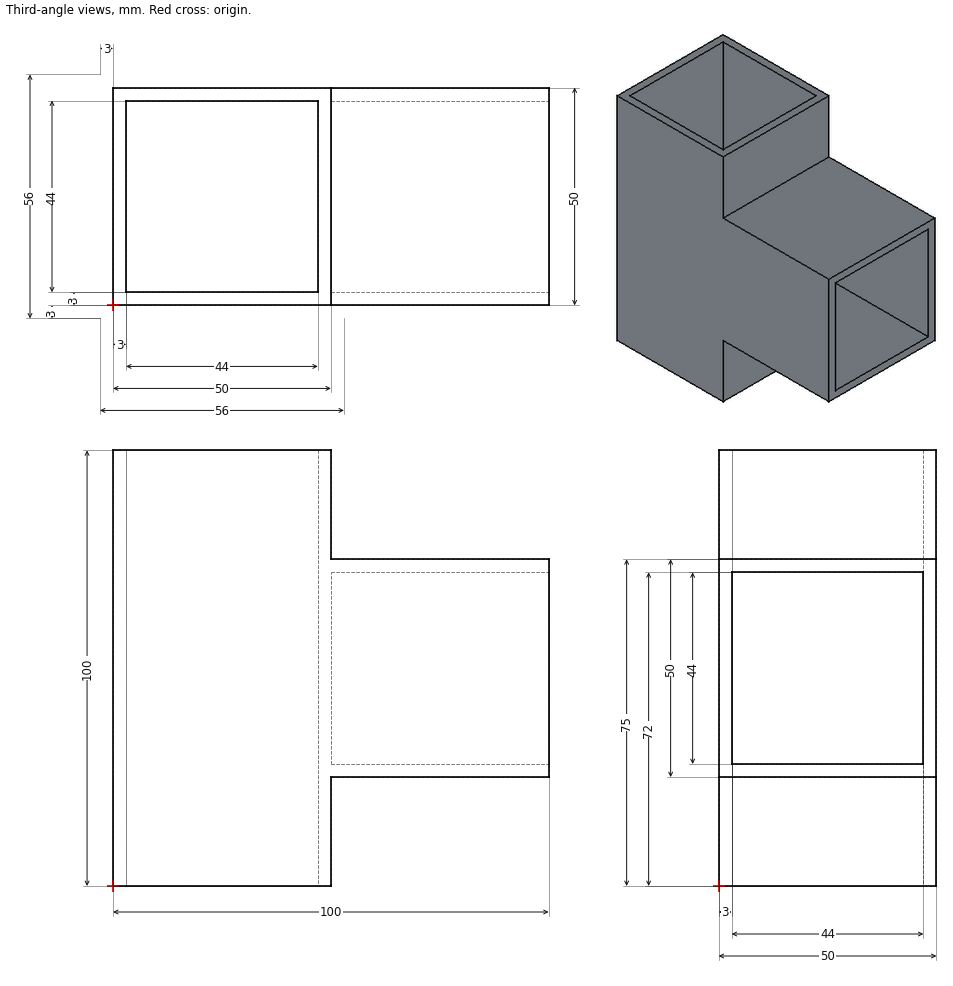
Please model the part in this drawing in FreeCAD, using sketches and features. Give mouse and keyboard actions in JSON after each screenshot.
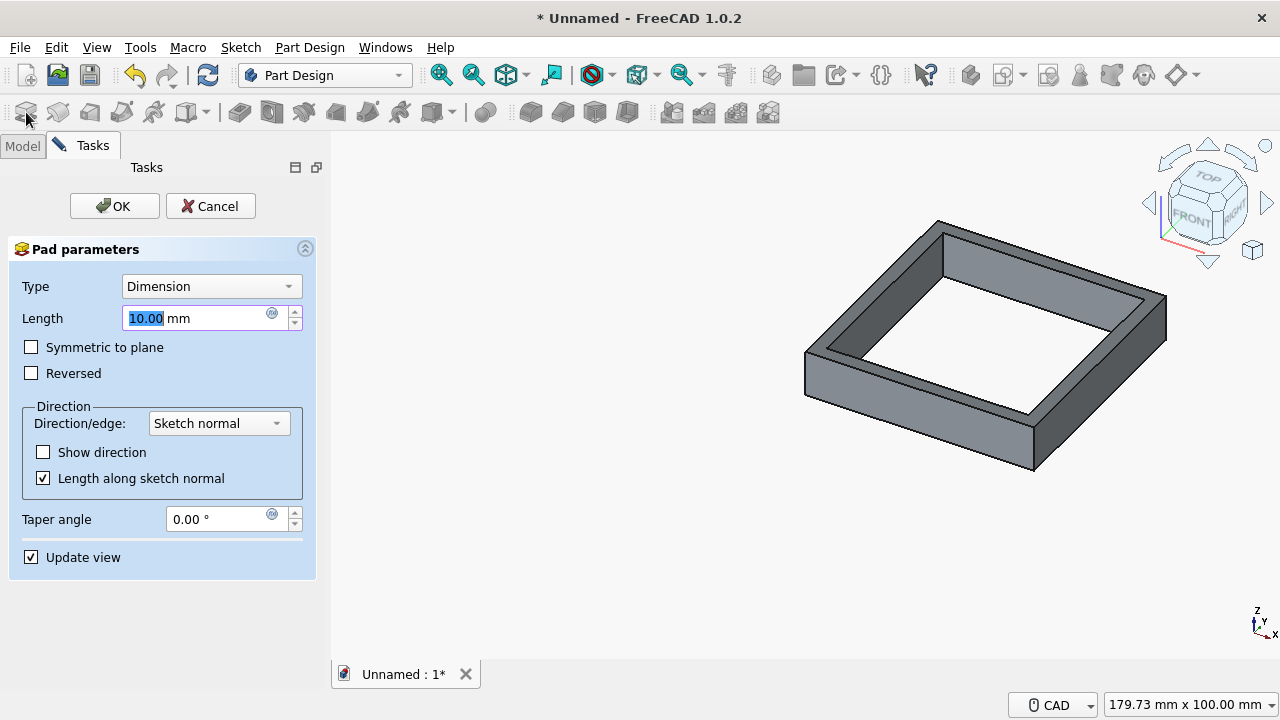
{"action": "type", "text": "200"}
{"action": "key", "text": "Tab"}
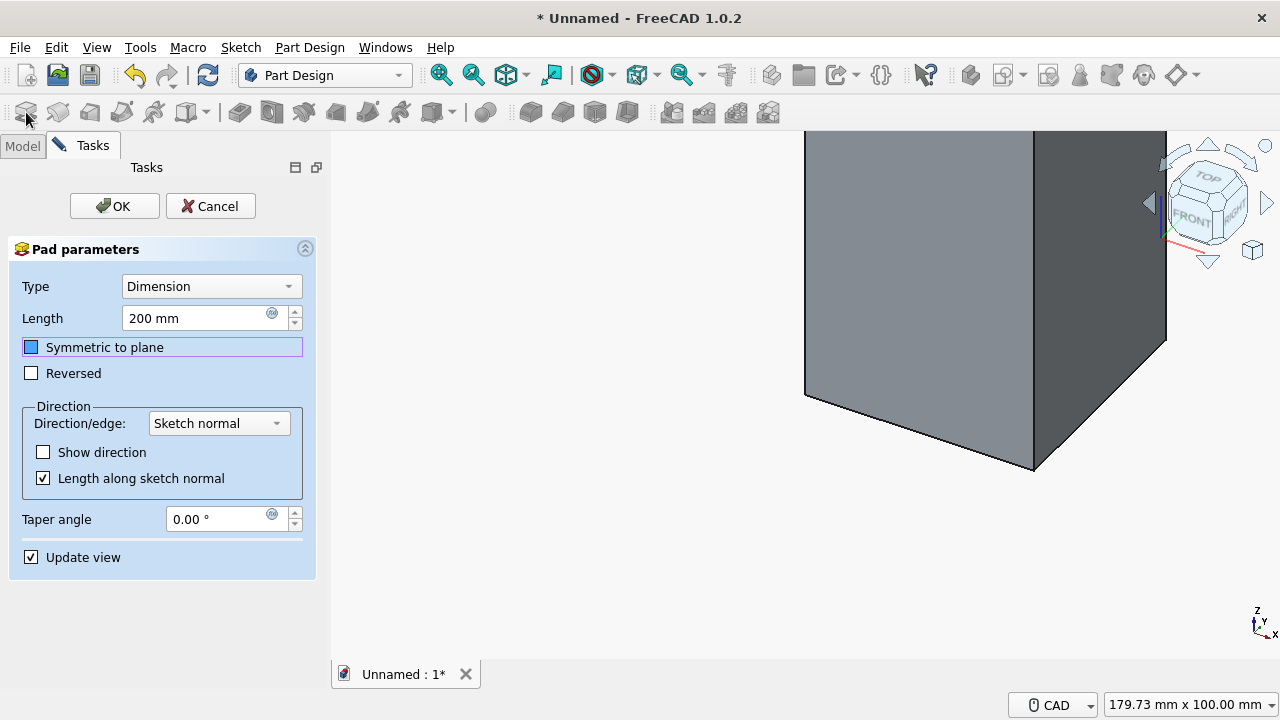
{"action": "left_click", "coordinate": [115, 206]}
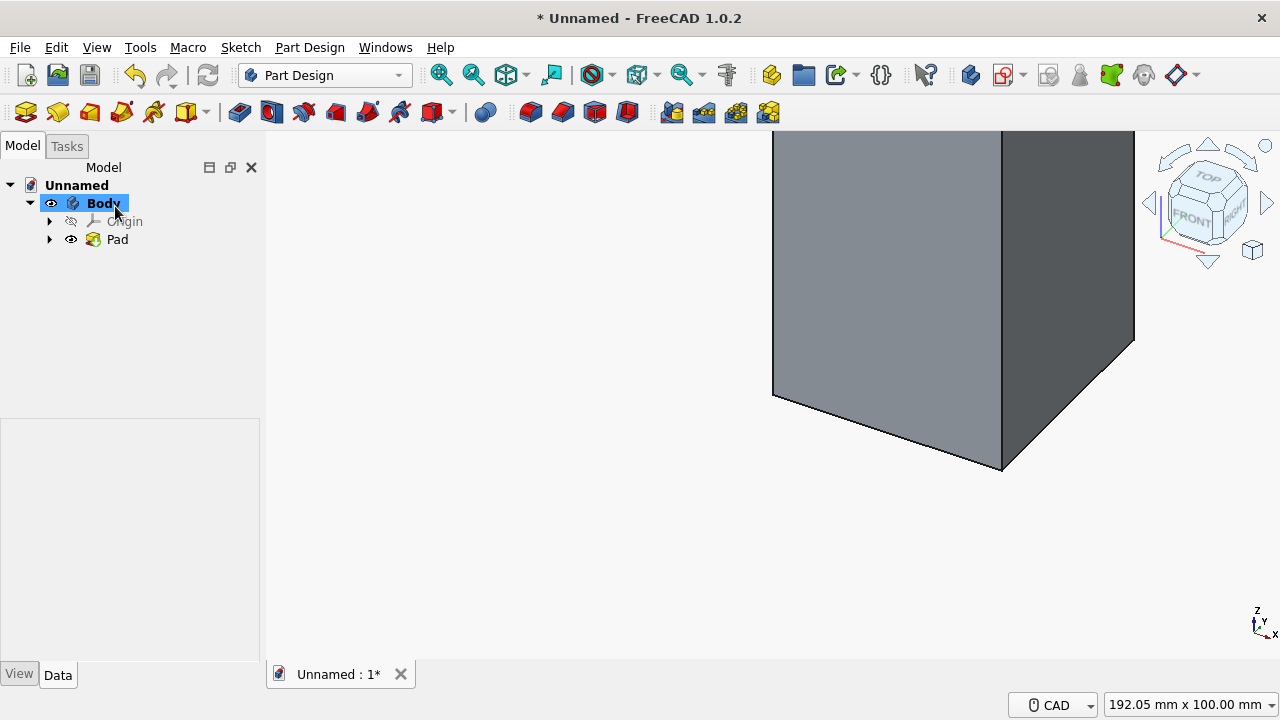
{"action": "key", "text": "v f"}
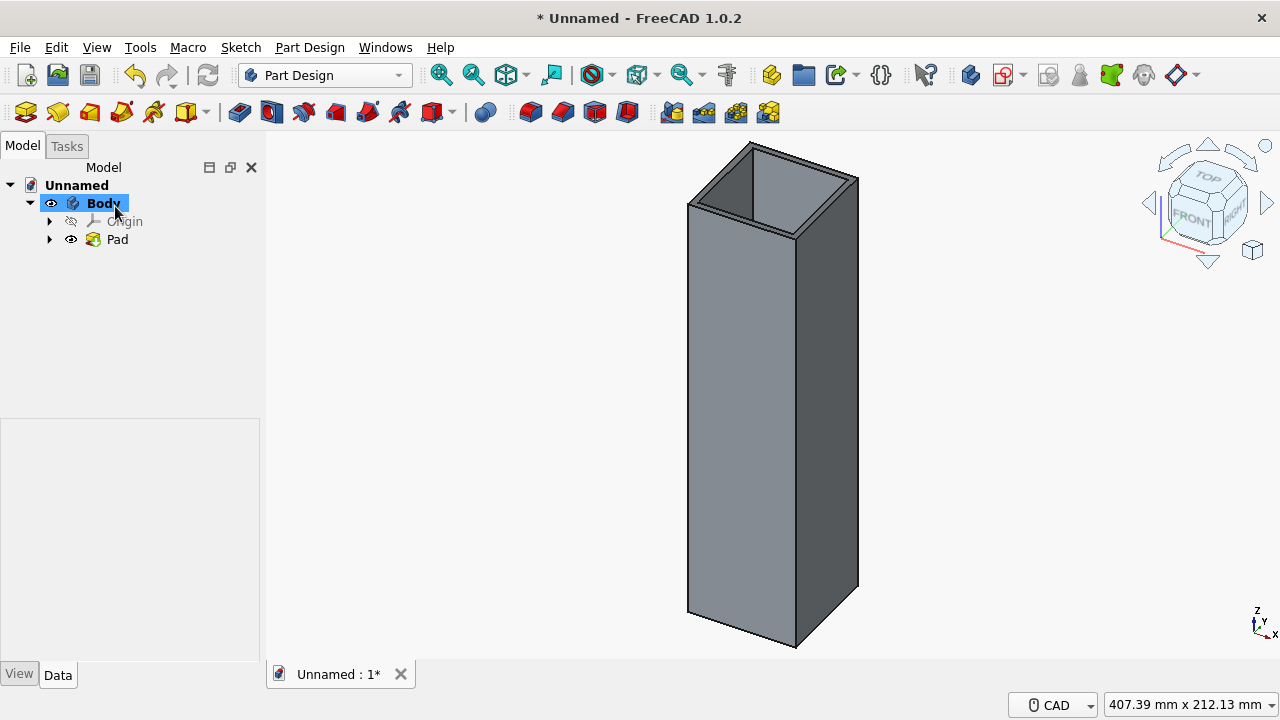
{"action": "scroll", "coordinate": [816, 216], "scroll_direction": "up", "scroll_amount": 8}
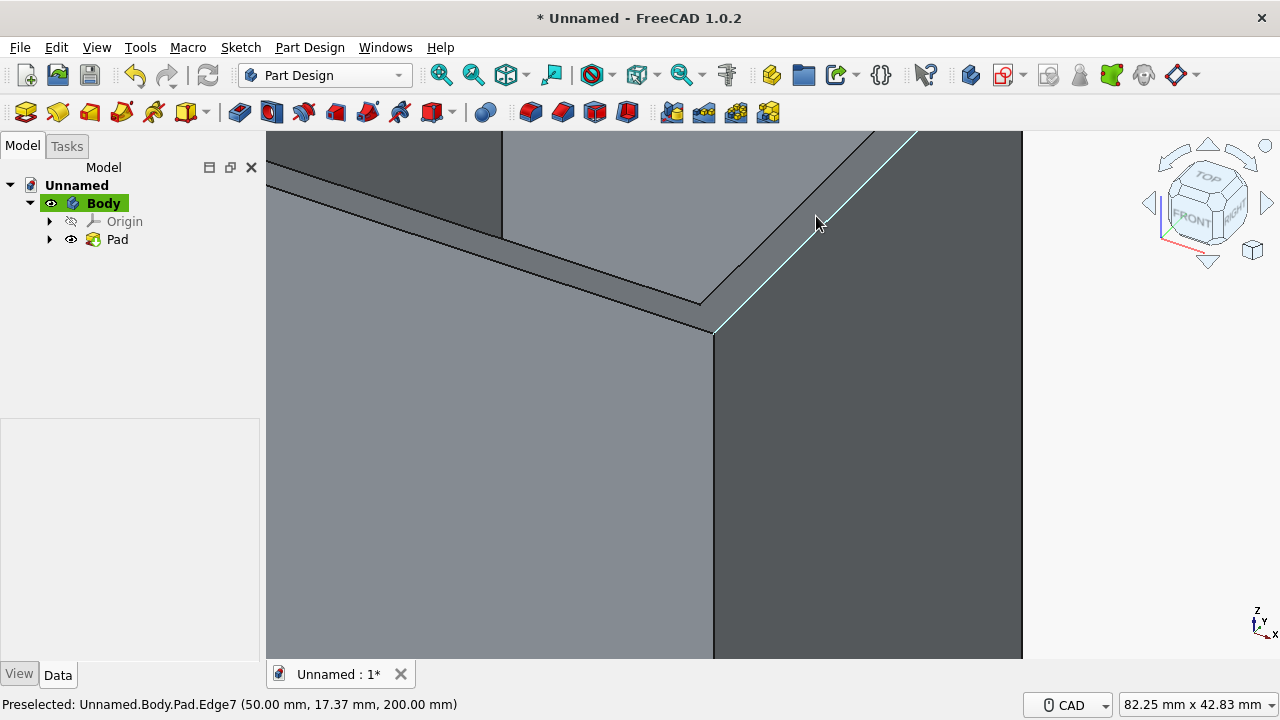
{"action": "left_click", "coordinate": [812, 221]}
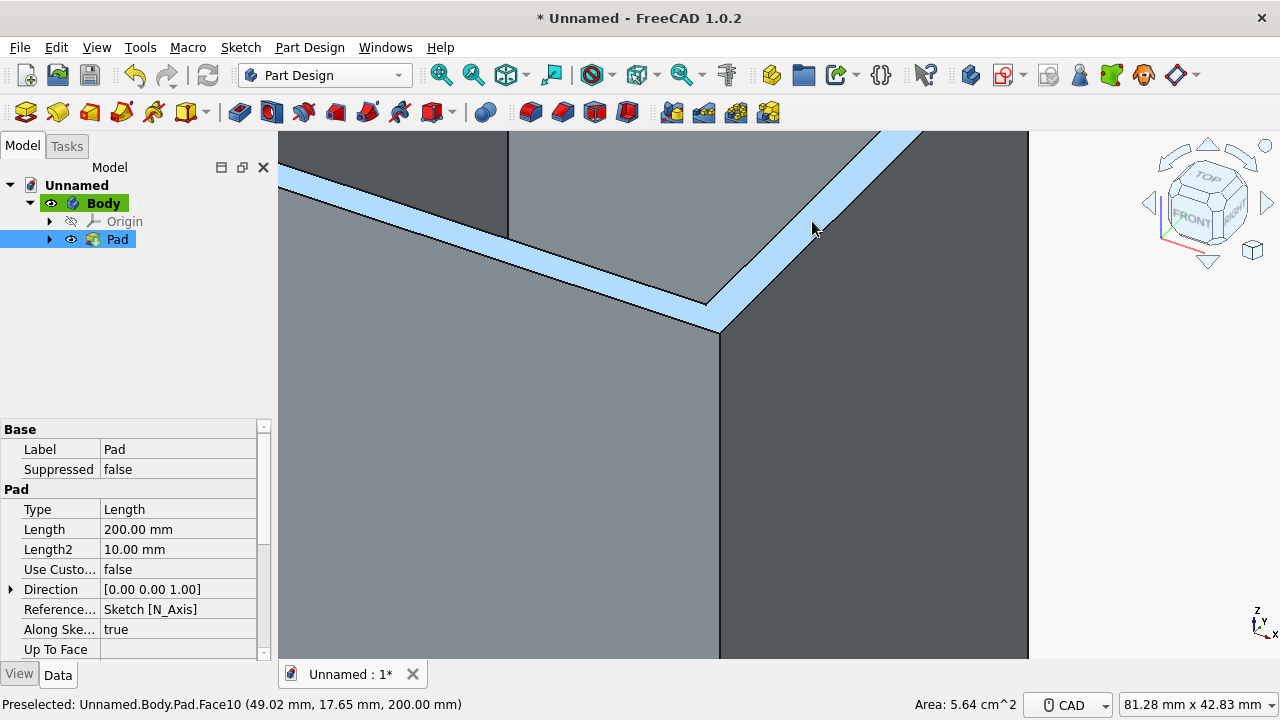
{"action": "left_click", "coordinate": [1004, 76]}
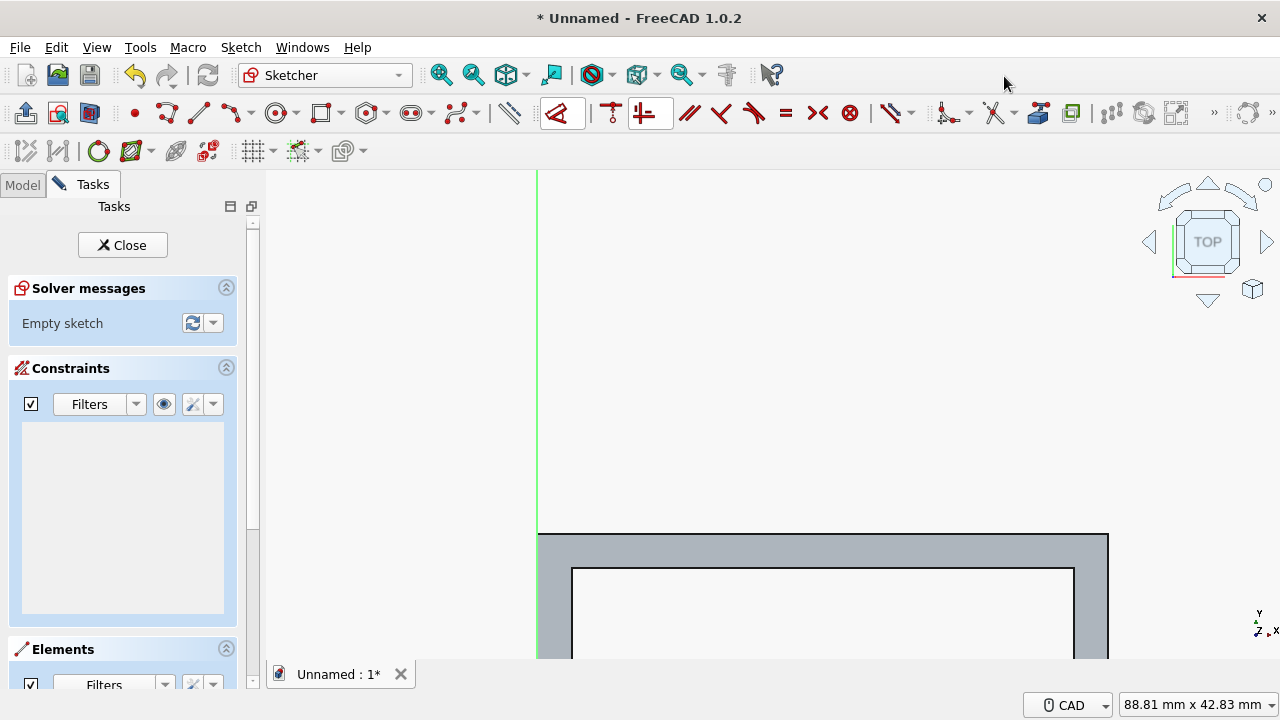
{"action": "scroll", "coordinate": [636, 198], "scroll_direction": "down", "scroll_amount": 5}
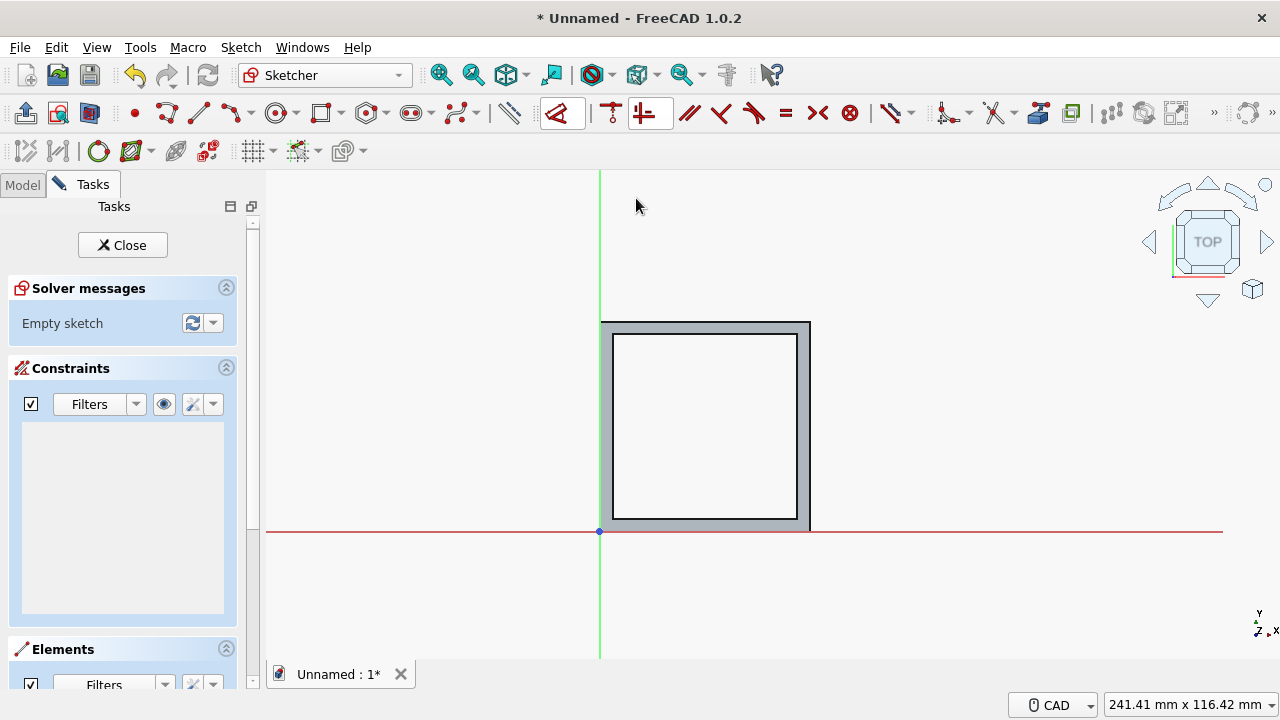
{"action": "left_click", "coordinate": [322, 114]}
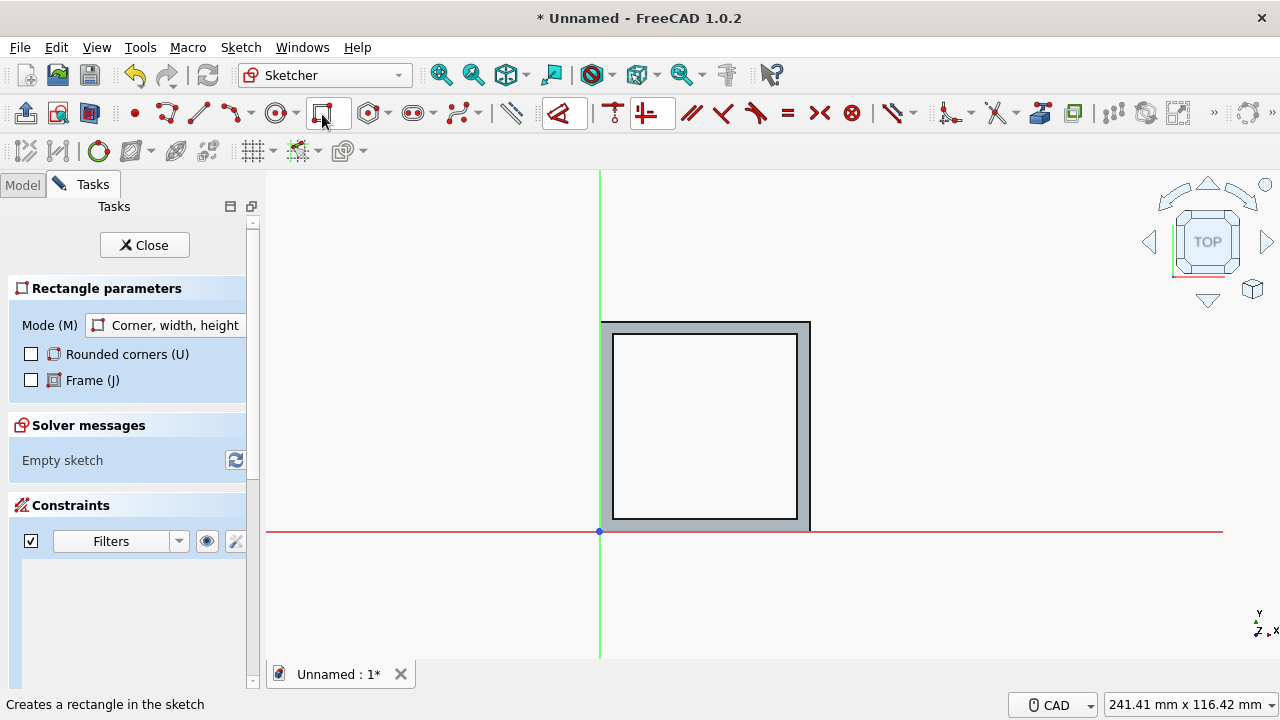
{"action": "scroll", "coordinate": [587, 309], "scroll_direction": "up", "scroll_amount": 2}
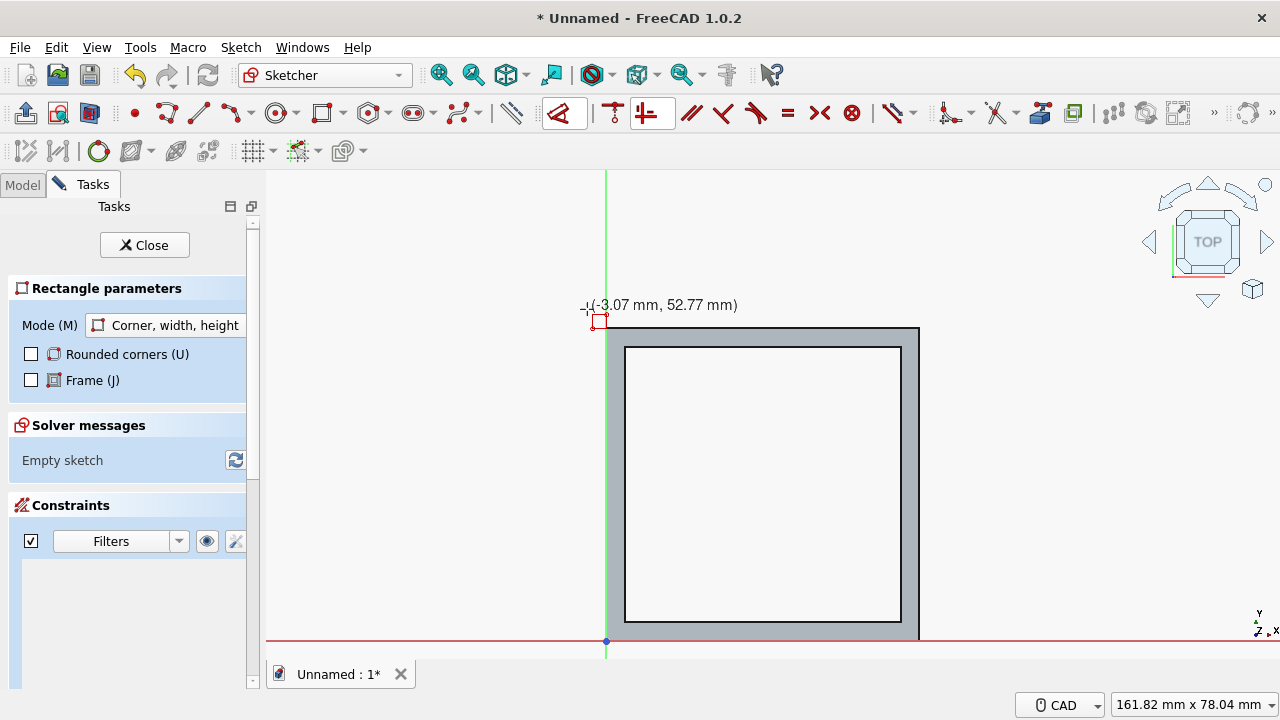
{"action": "left_click", "coordinate": [587, 309]}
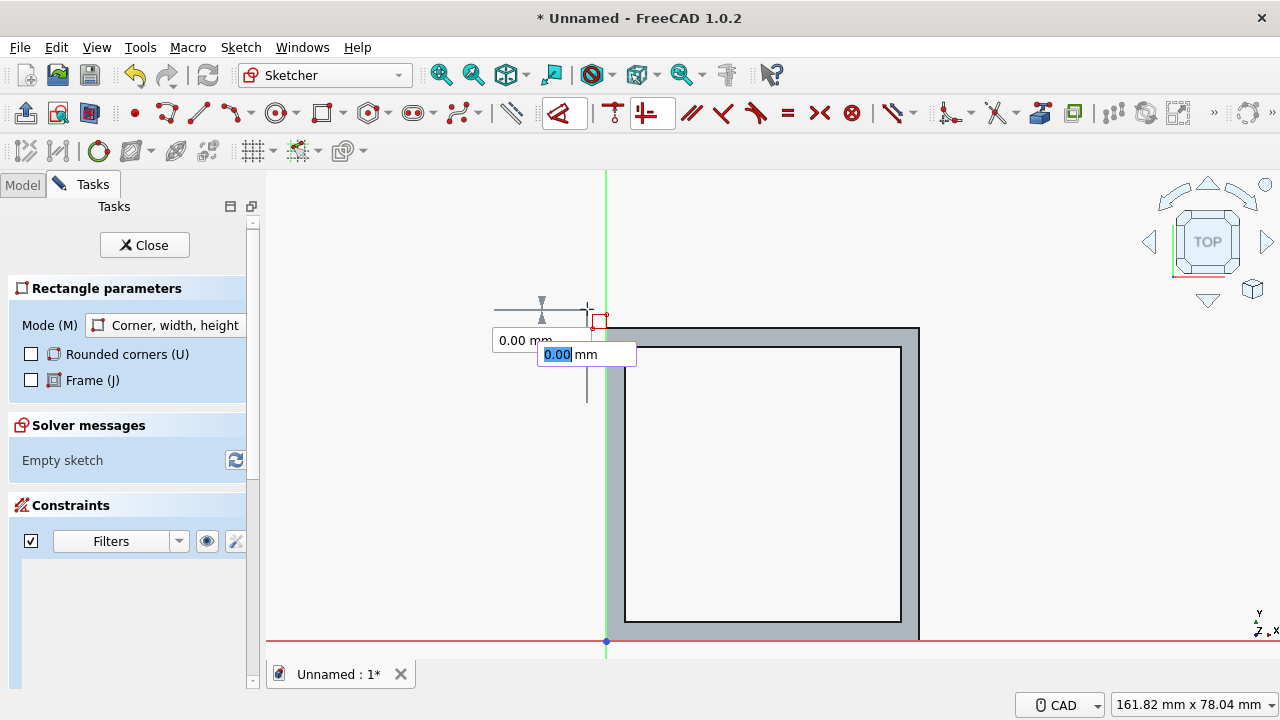
{"action": "scroll", "coordinate": [441, 198], "scroll_direction": "down", "scroll_amount": 1}